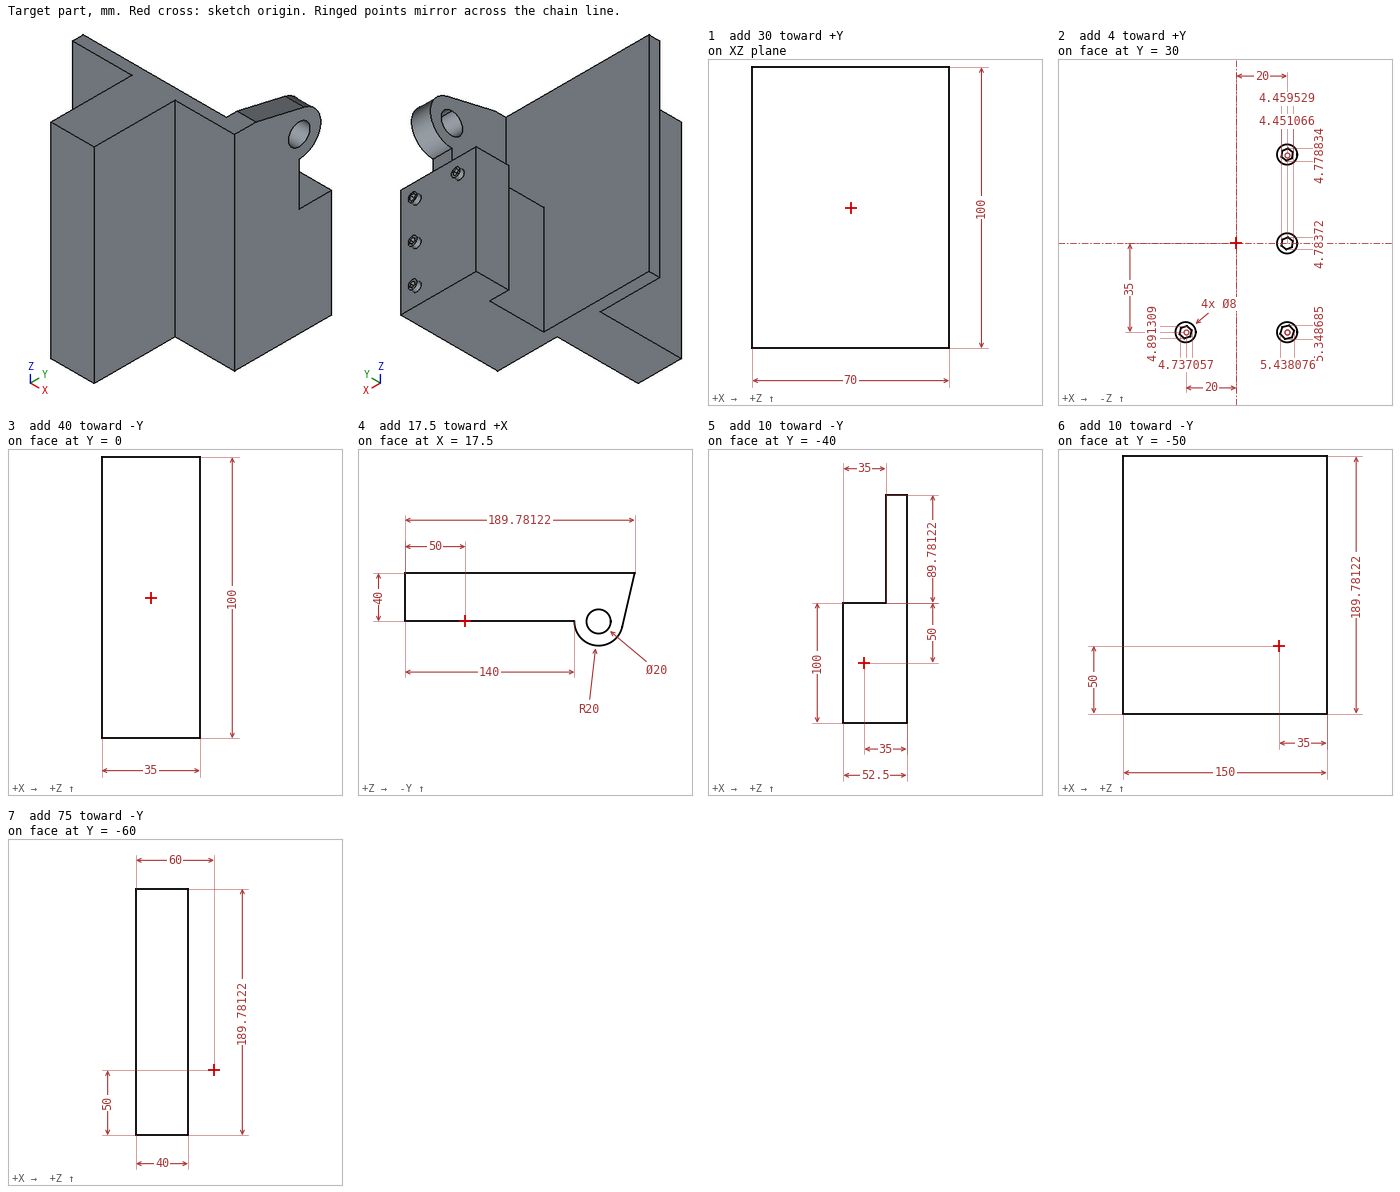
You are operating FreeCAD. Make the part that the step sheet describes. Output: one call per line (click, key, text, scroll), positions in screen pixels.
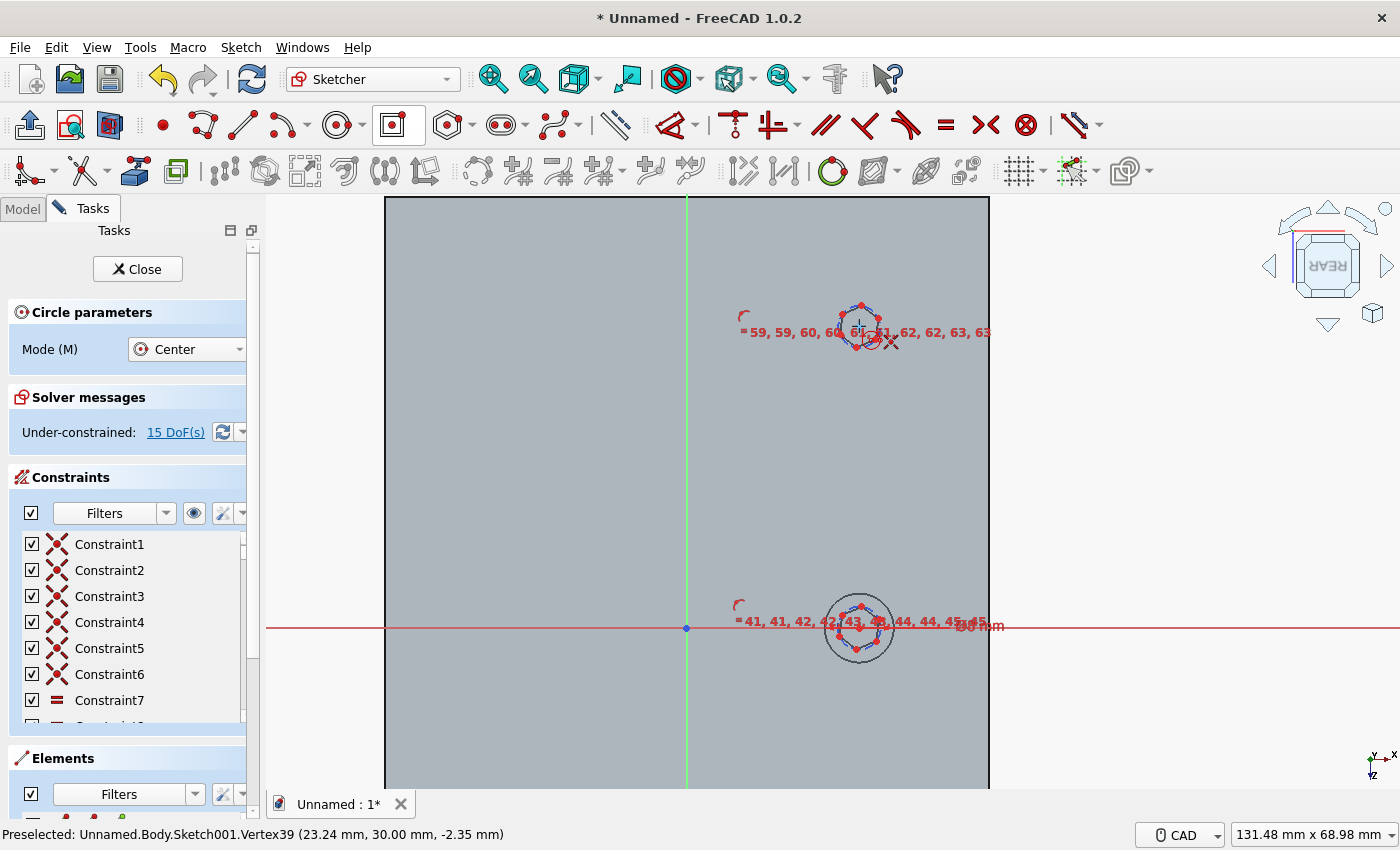
click(859, 327)
move(884, 302)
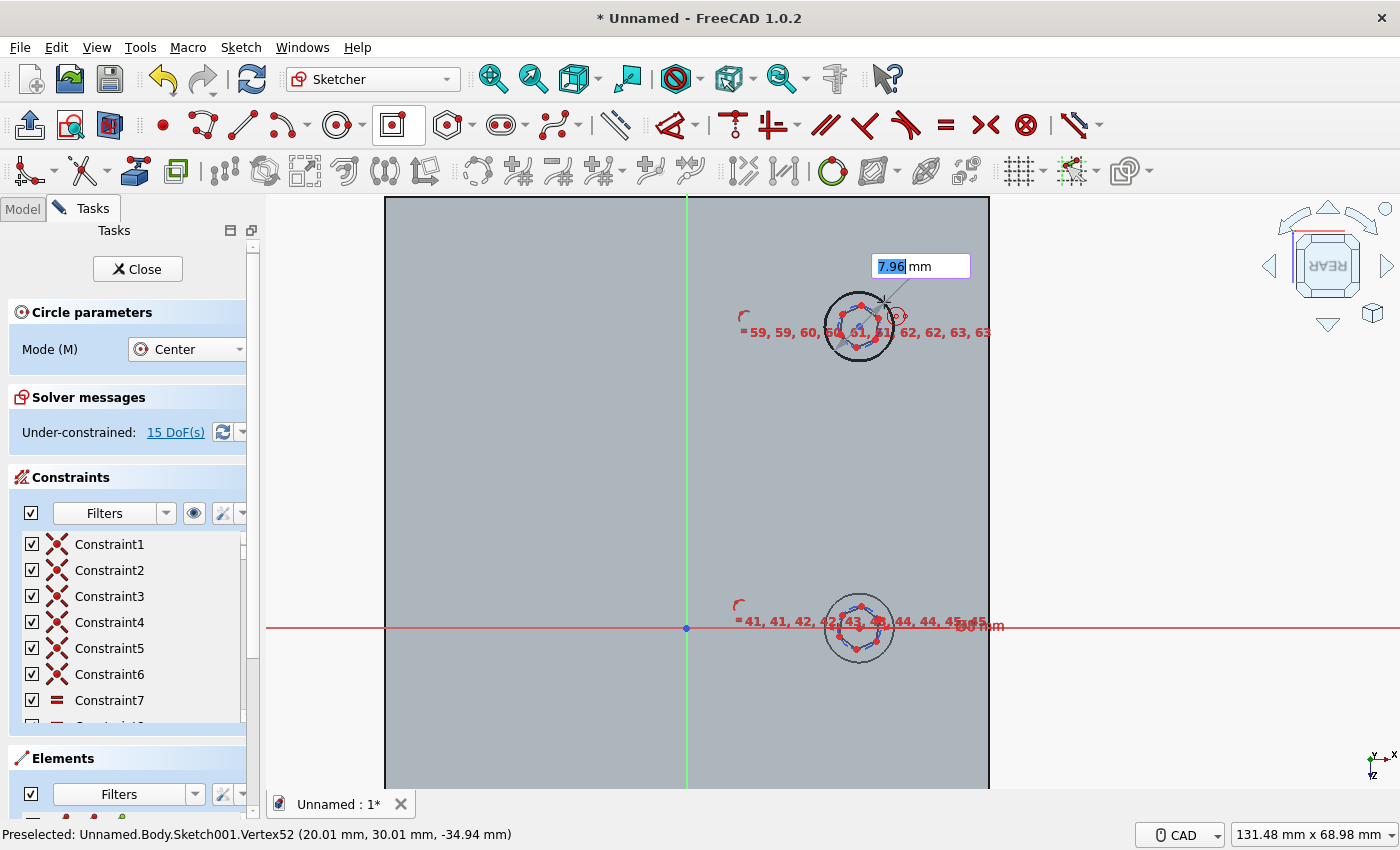
text(8)
key(Return)
key(Escape)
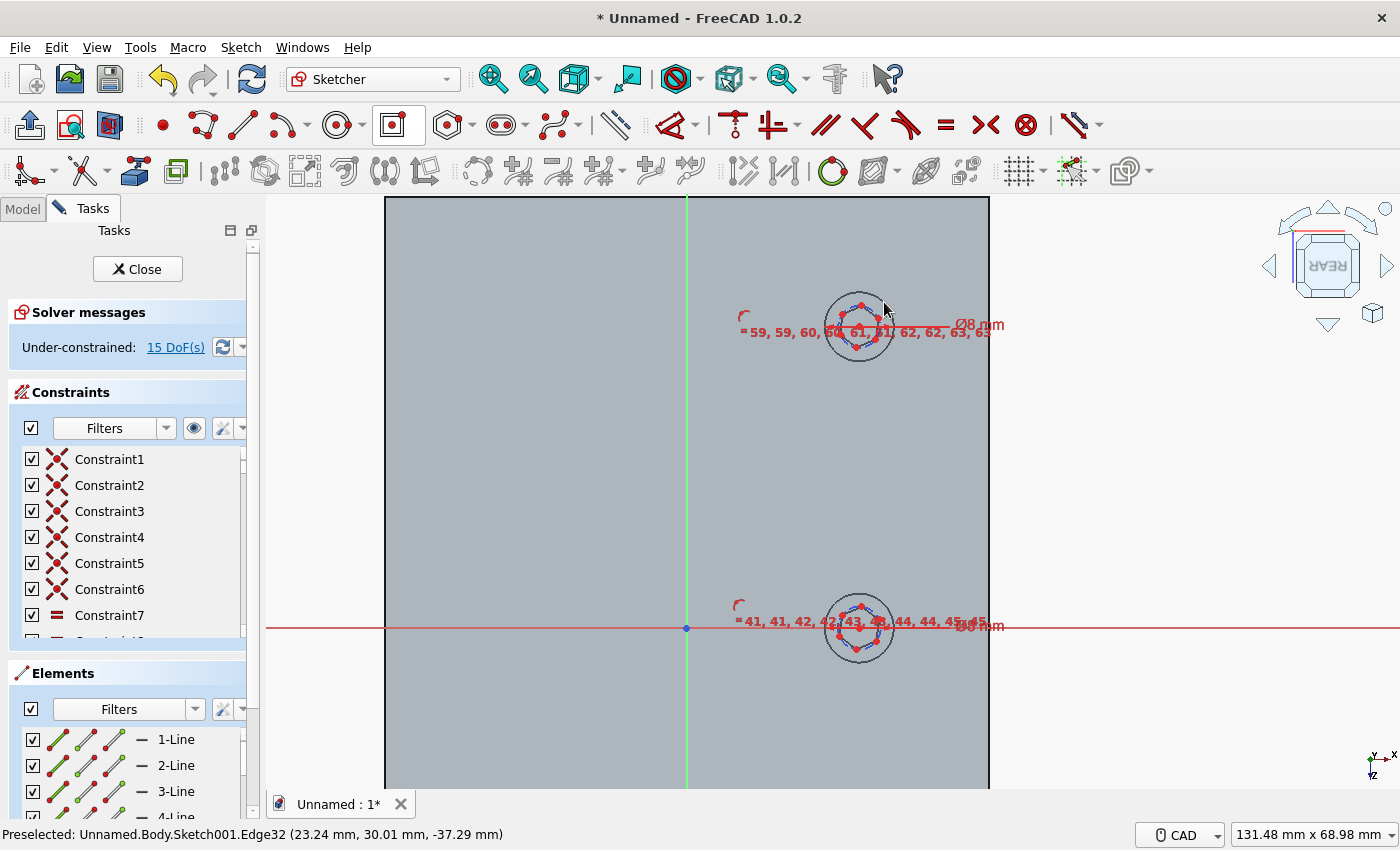
scroll(859, 325, down, 3)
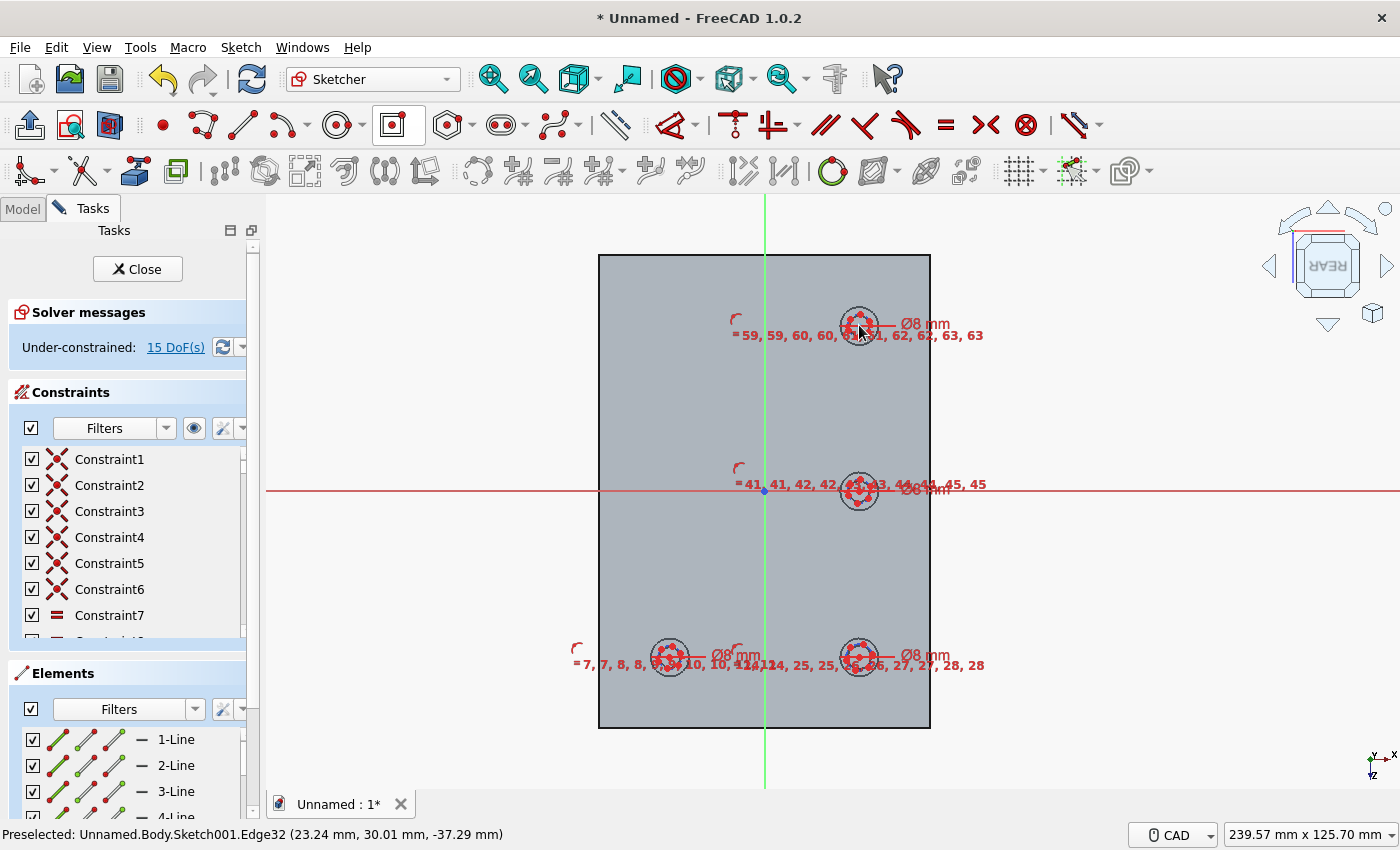
click(670, 657)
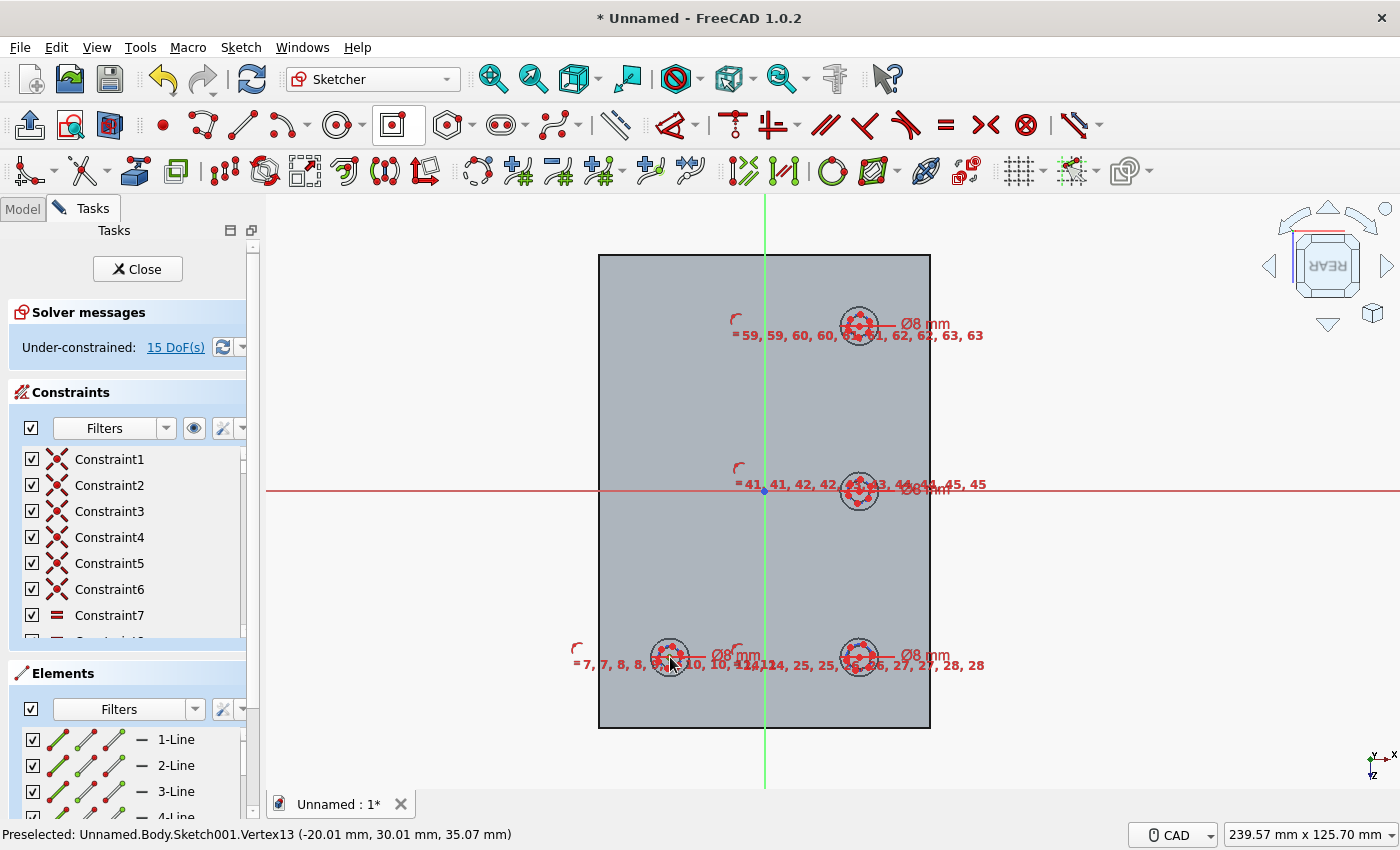
click(859, 657)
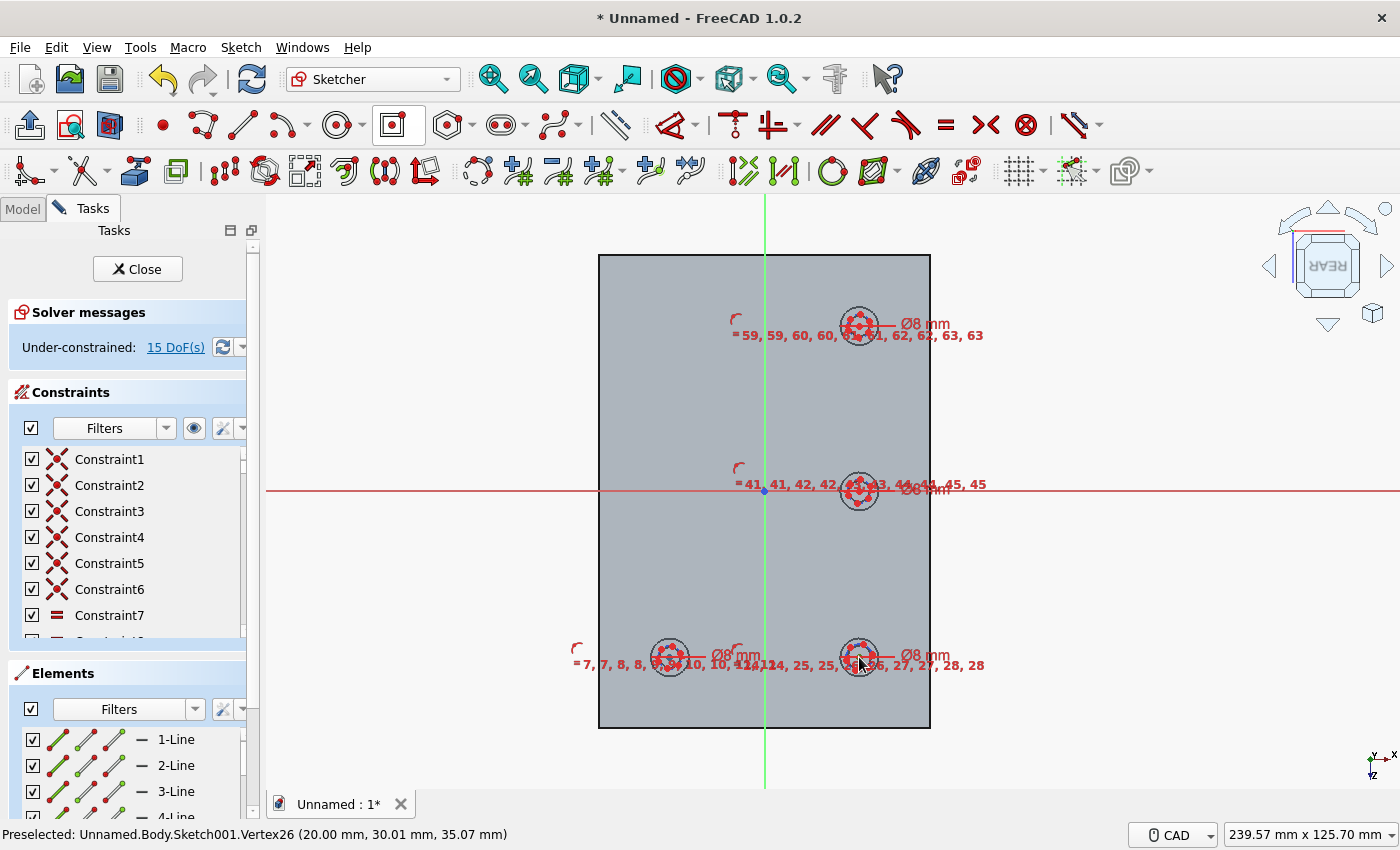
click(765, 722)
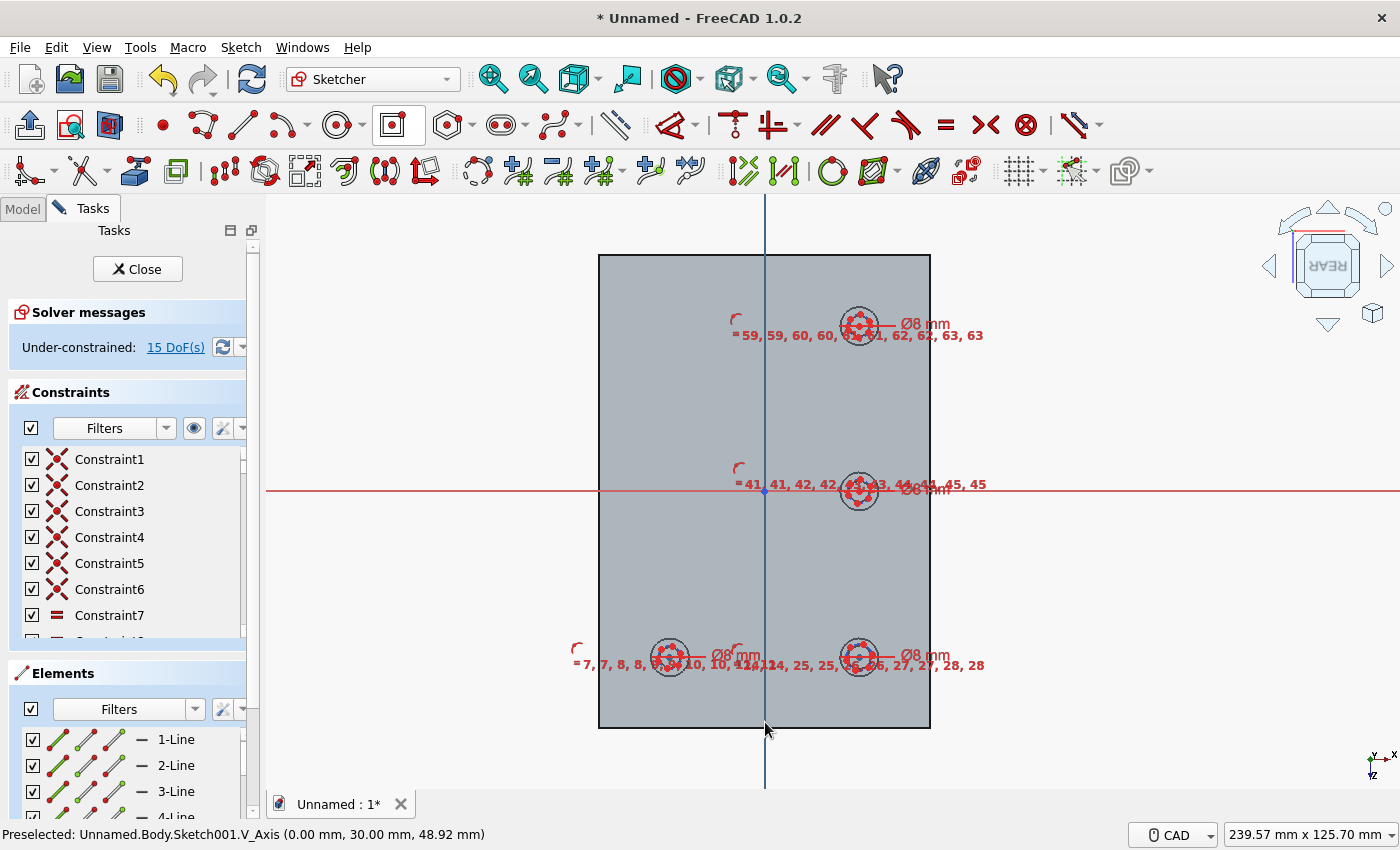
click(986, 126)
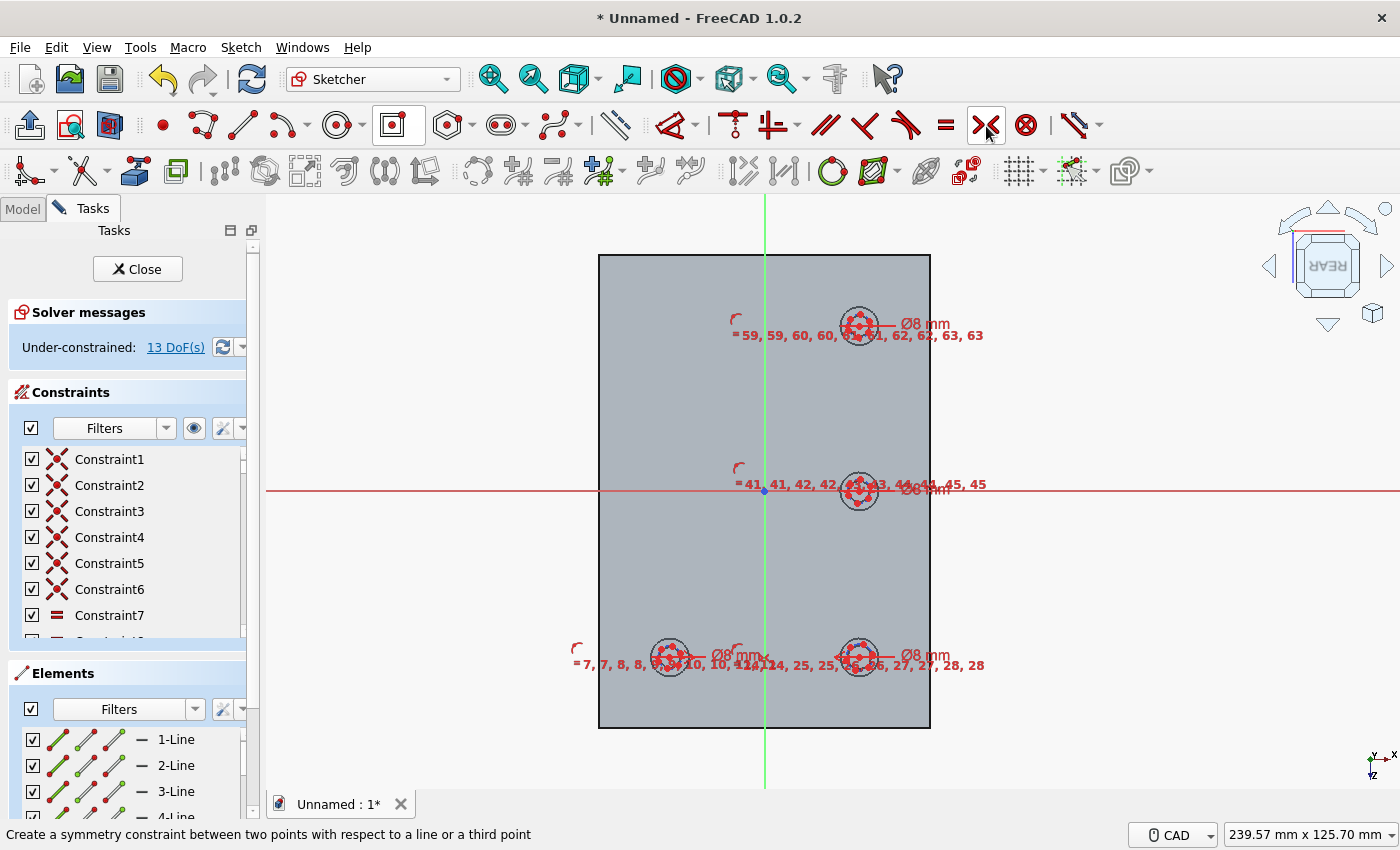
click(859, 657)